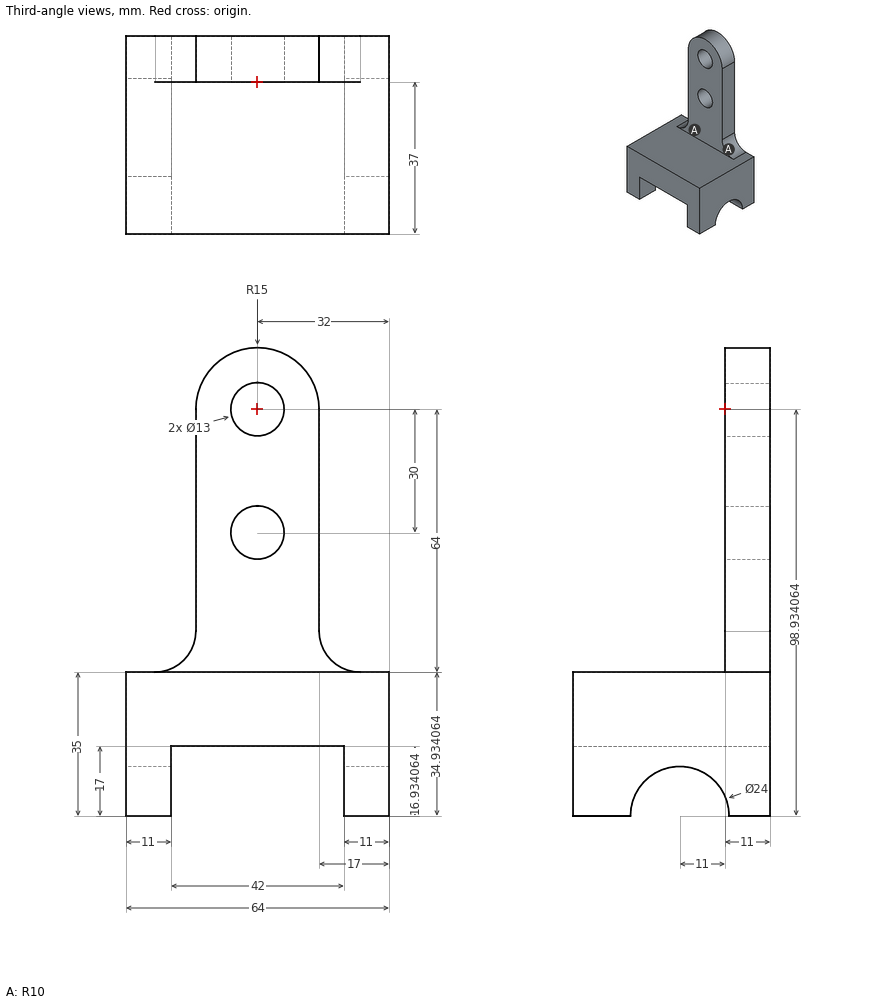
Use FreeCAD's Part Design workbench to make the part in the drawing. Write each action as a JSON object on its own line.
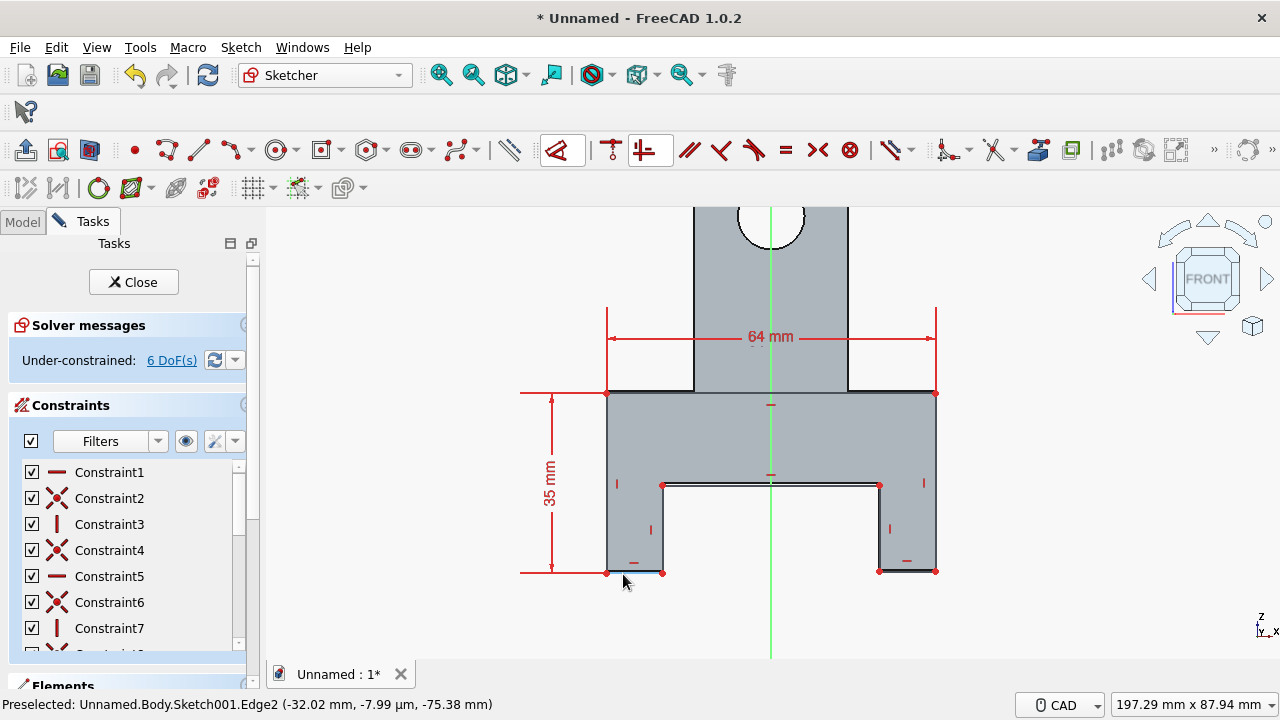
{"action": "left_click", "coordinate": [624, 573]}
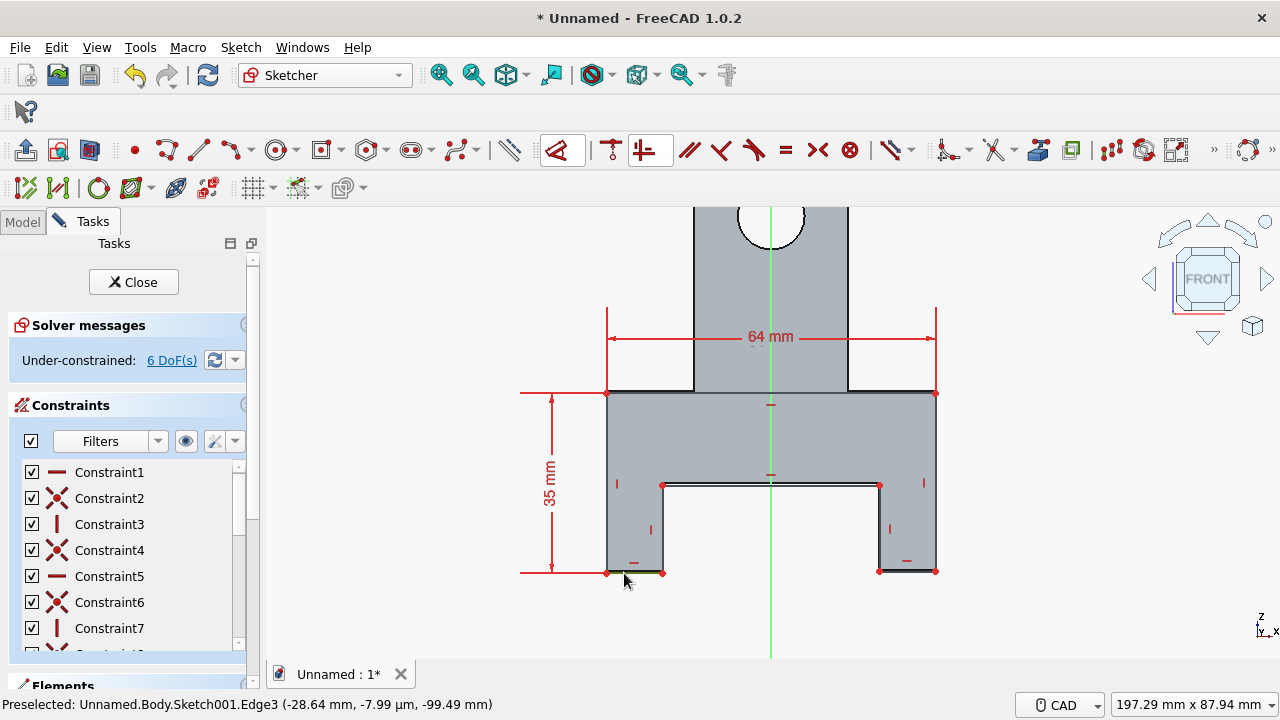
{"action": "key", "text": "l"}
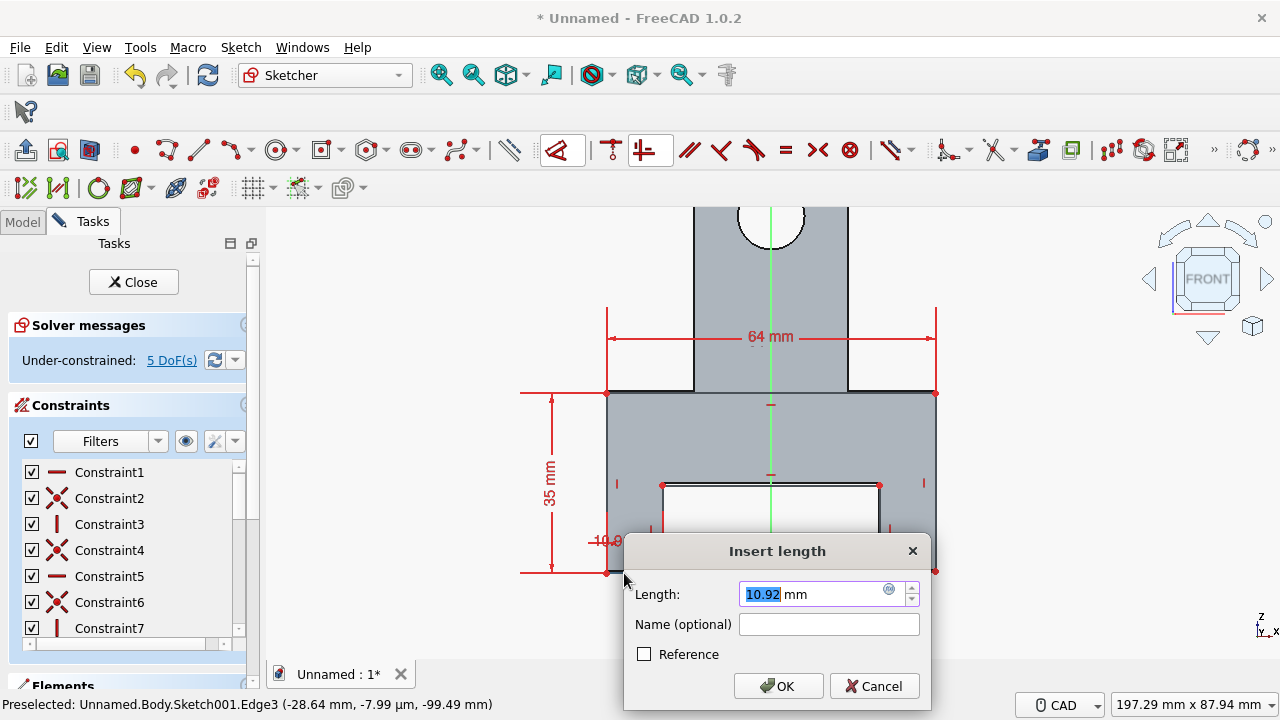
{"action": "type", "text": "11"}
{"action": "key", "text": "Return"}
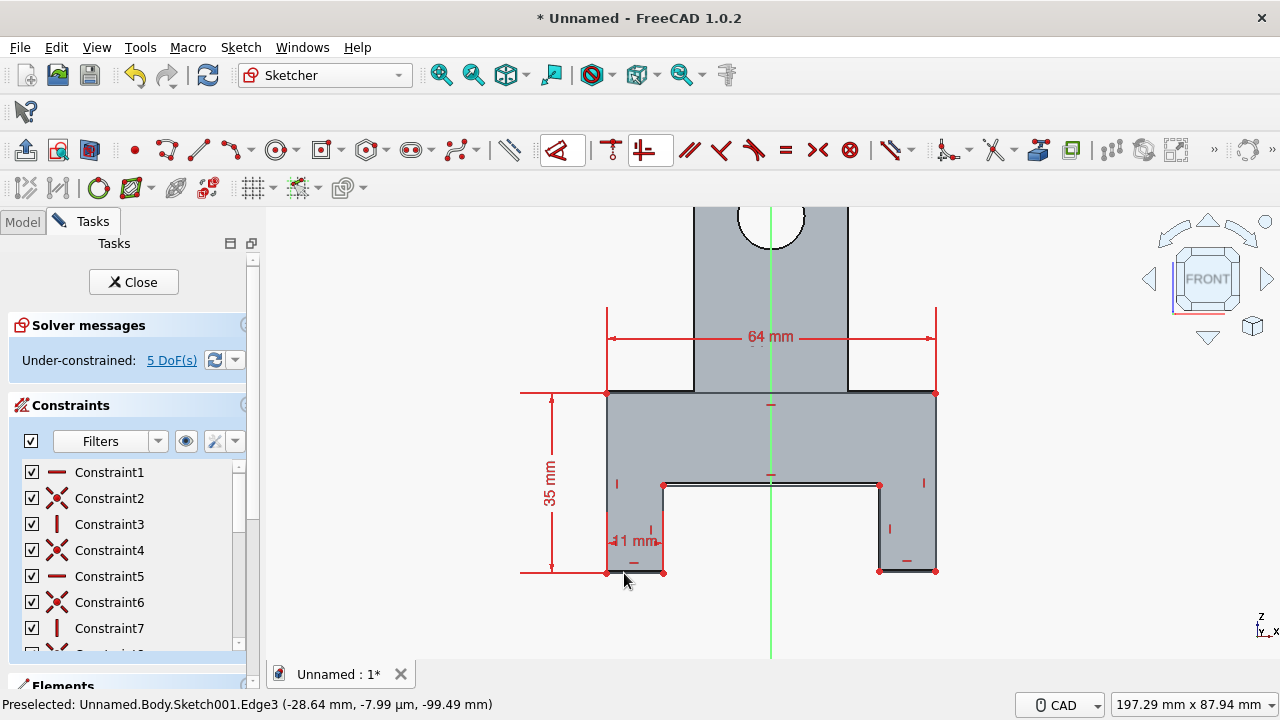
{"action": "left_click", "coordinate": [663, 547]}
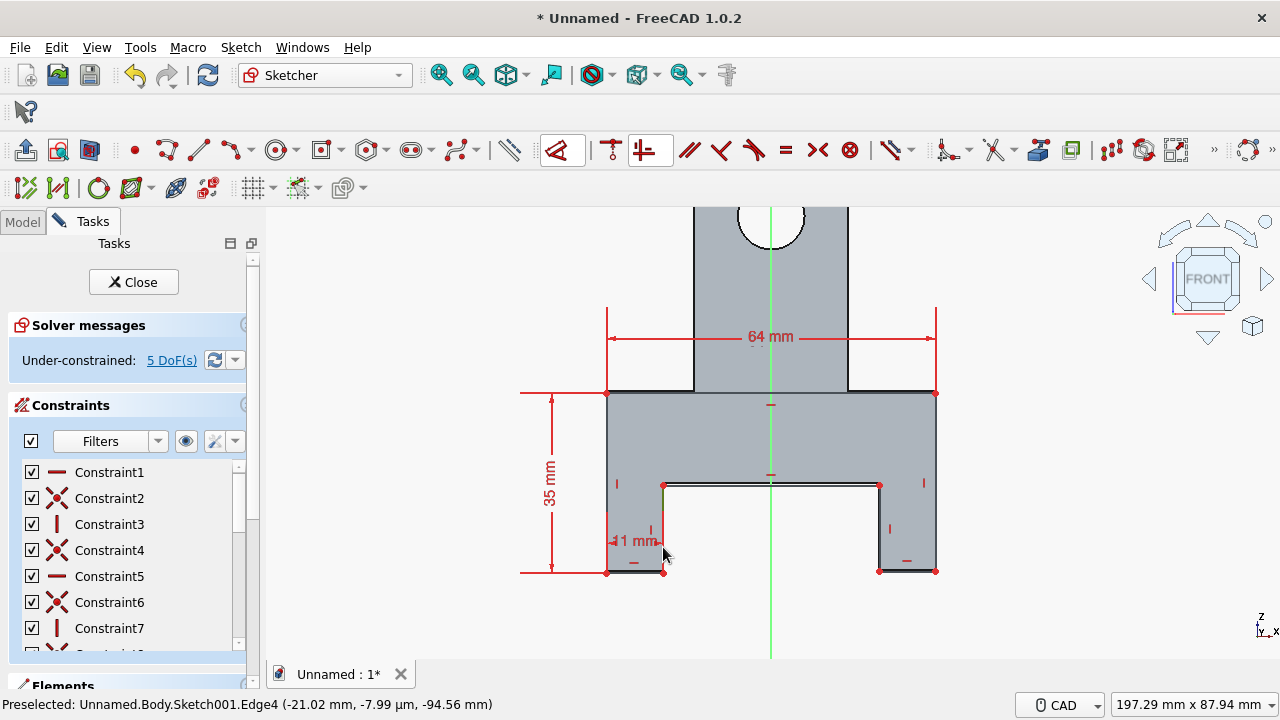
{"action": "key", "text": "i"}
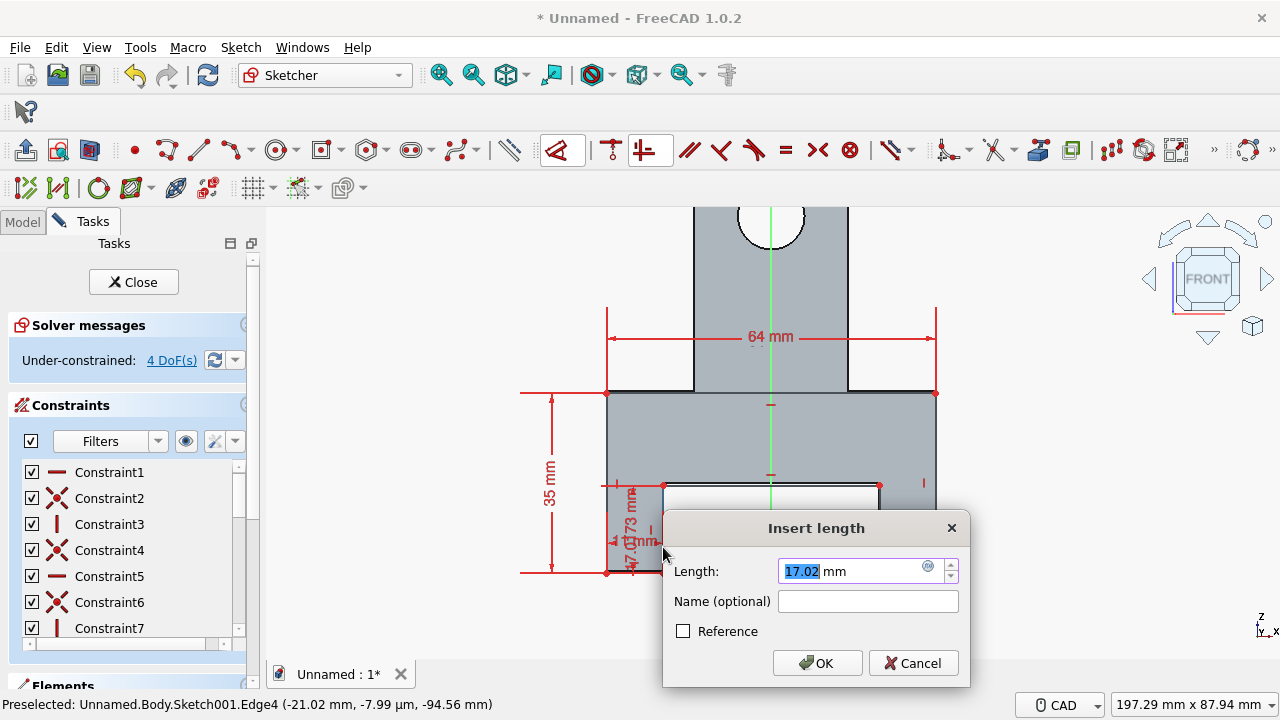
{"action": "type", "text": "17"}
{"action": "key", "text": "Return"}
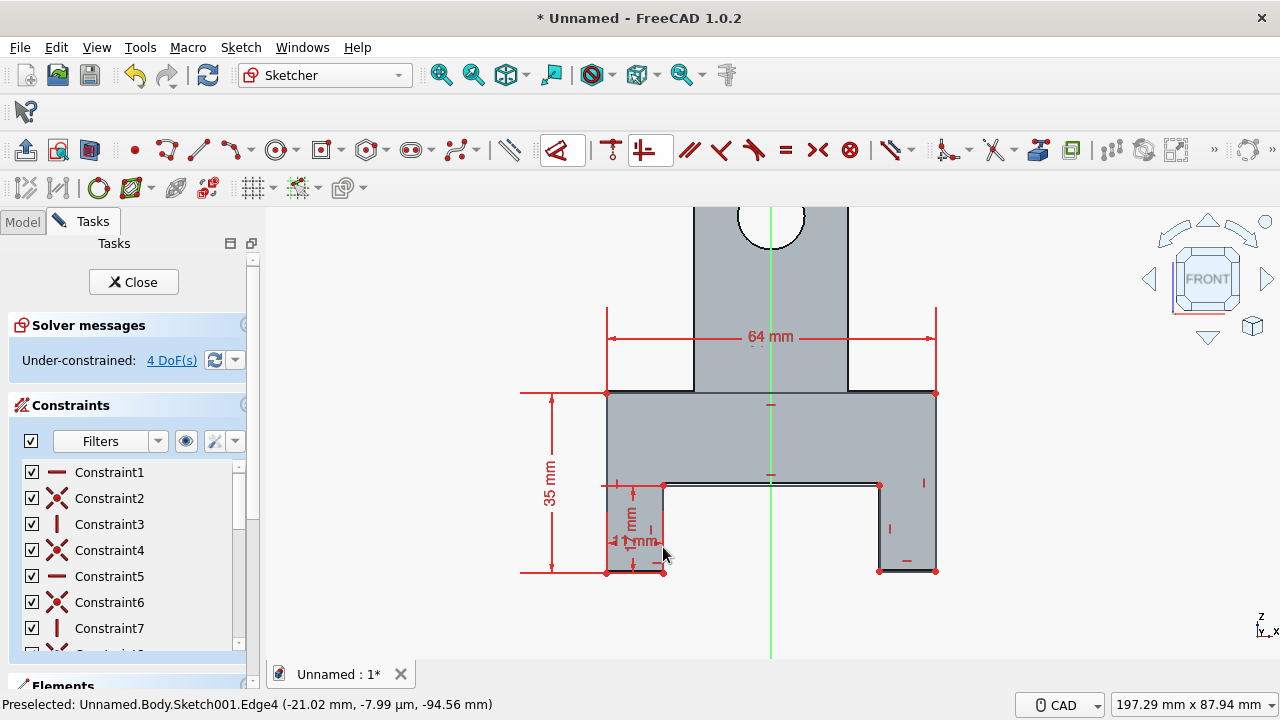
{"action": "left_click", "coordinate": [728, 486]}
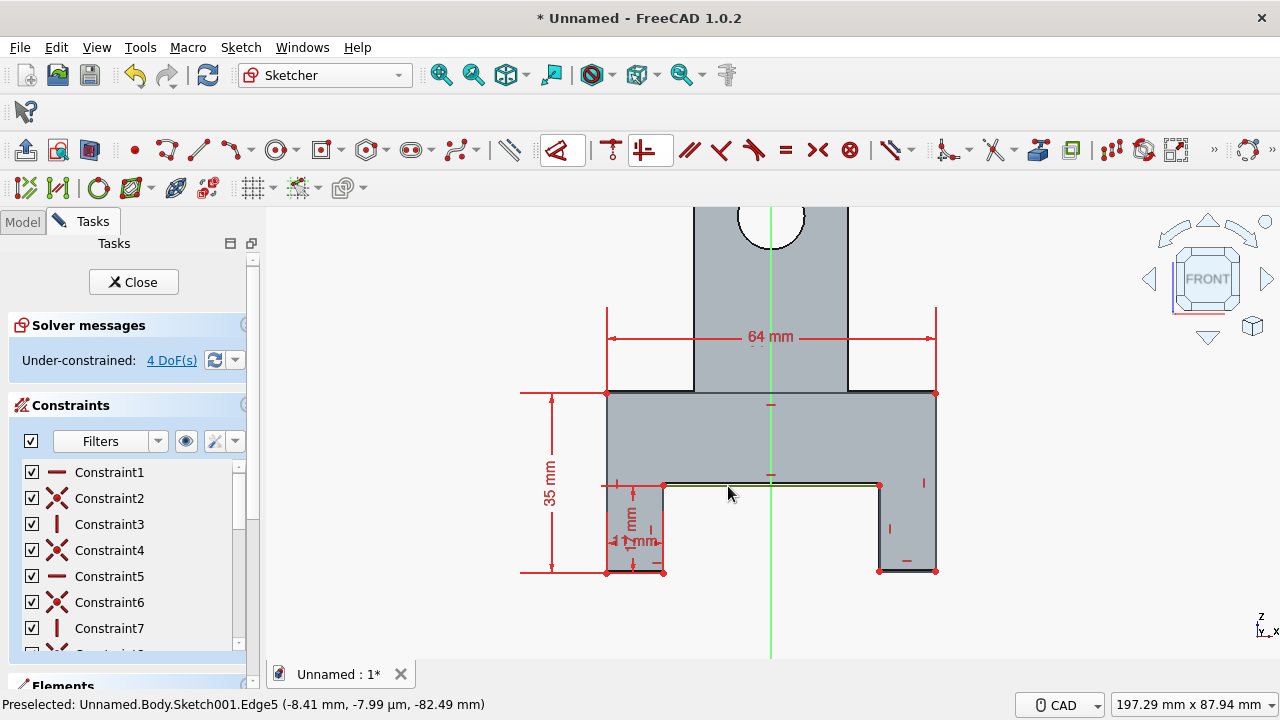
{"action": "left_click", "coordinate": [580, 150]}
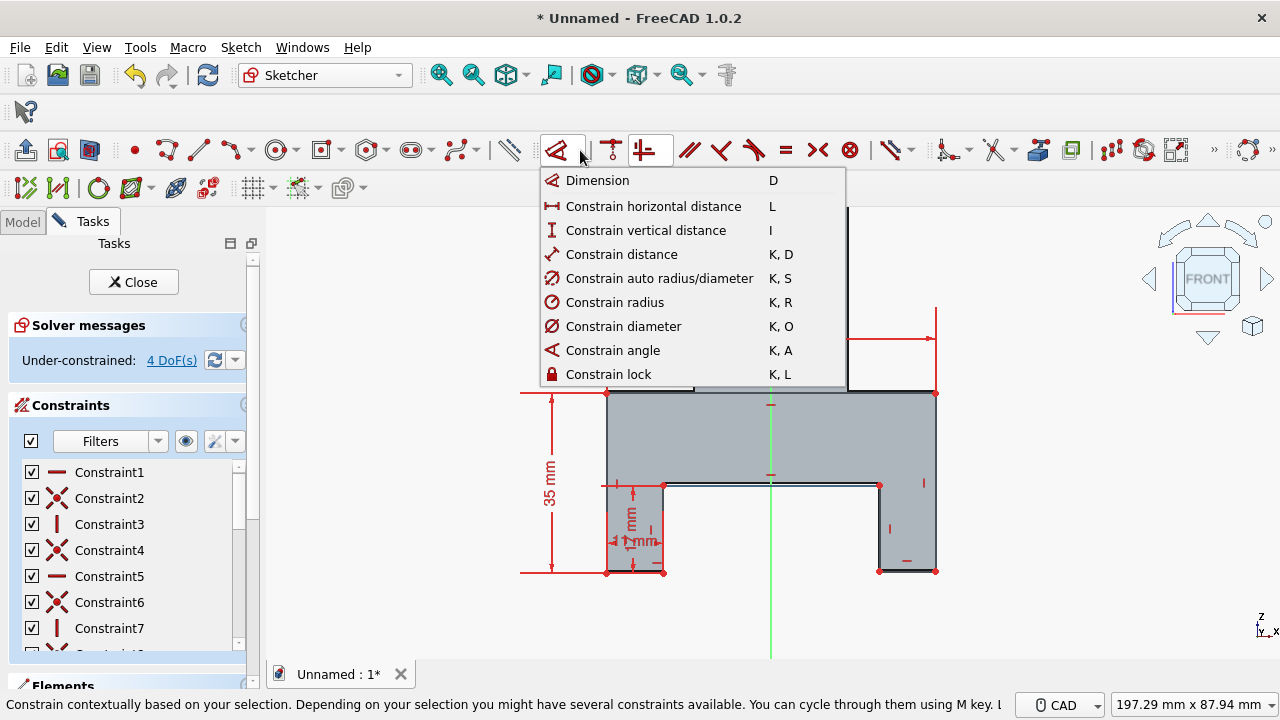
{"action": "left_click", "coordinate": [693, 206]}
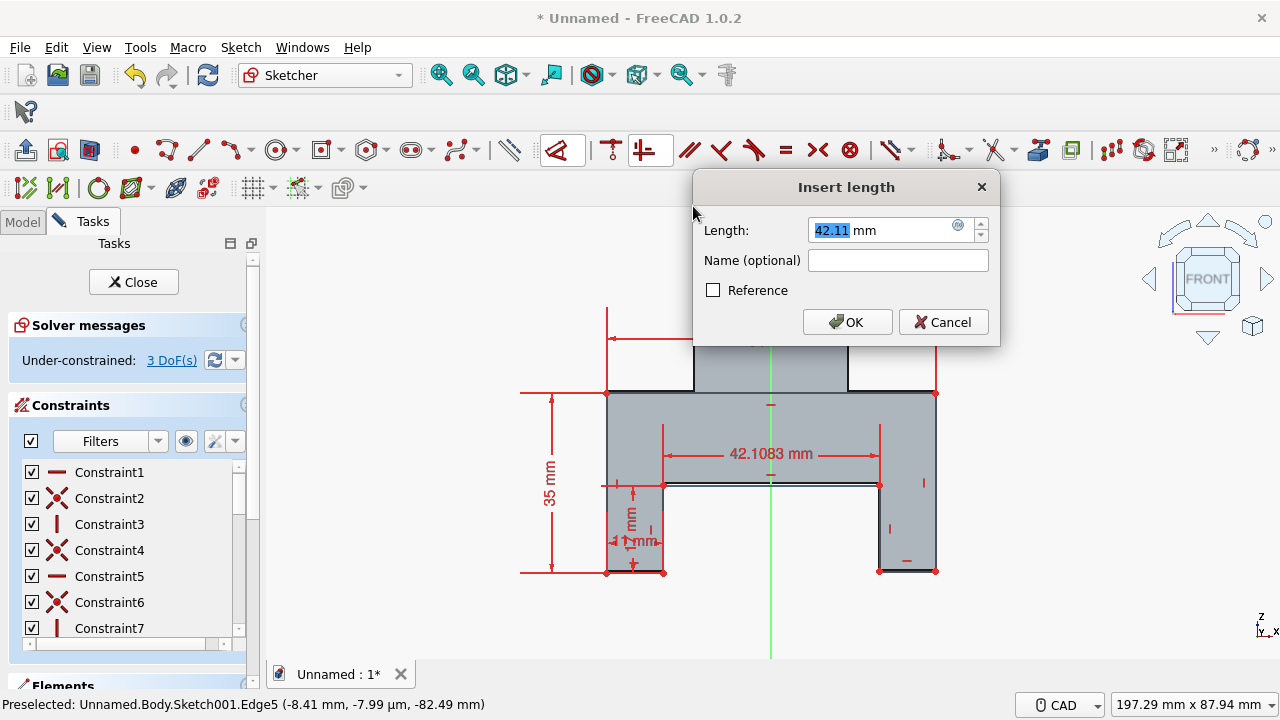
{"action": "type", "text": "42"}
{"action": "key", "text": "Return"}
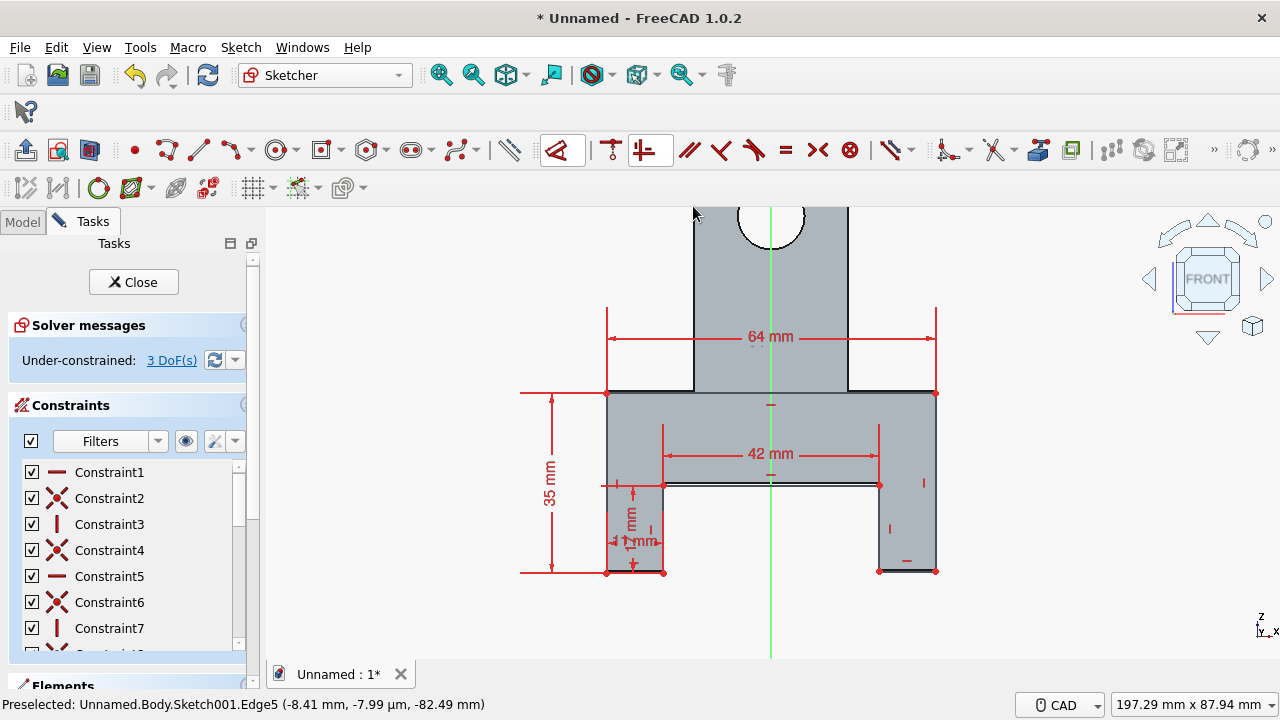
{"action": "left_click", "coordinate": [936, 393]}